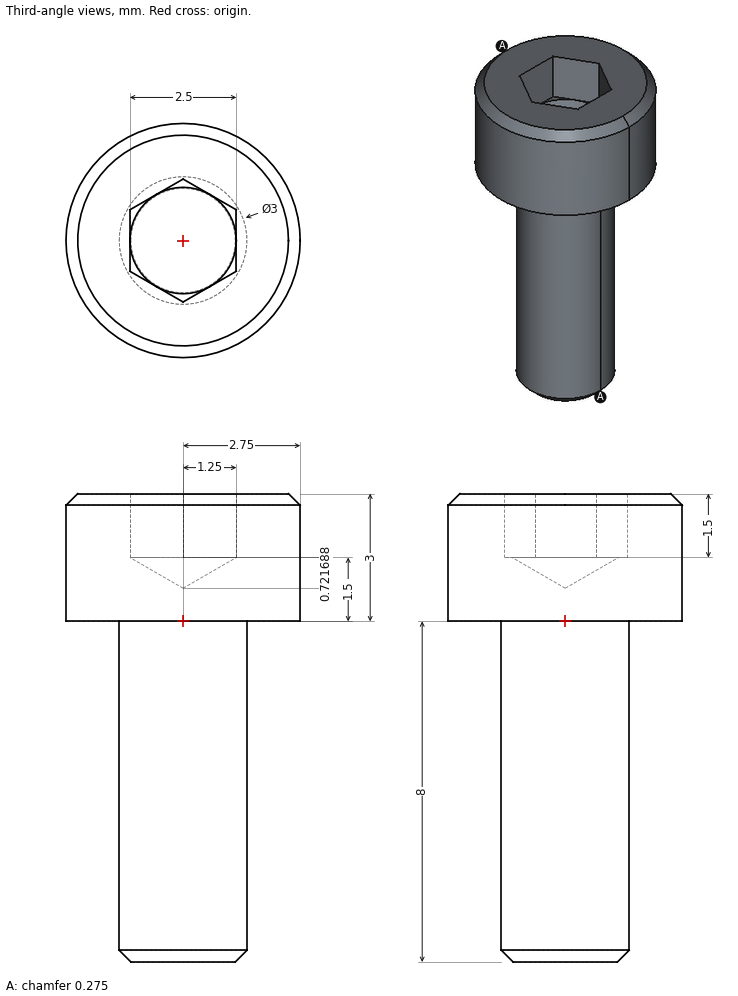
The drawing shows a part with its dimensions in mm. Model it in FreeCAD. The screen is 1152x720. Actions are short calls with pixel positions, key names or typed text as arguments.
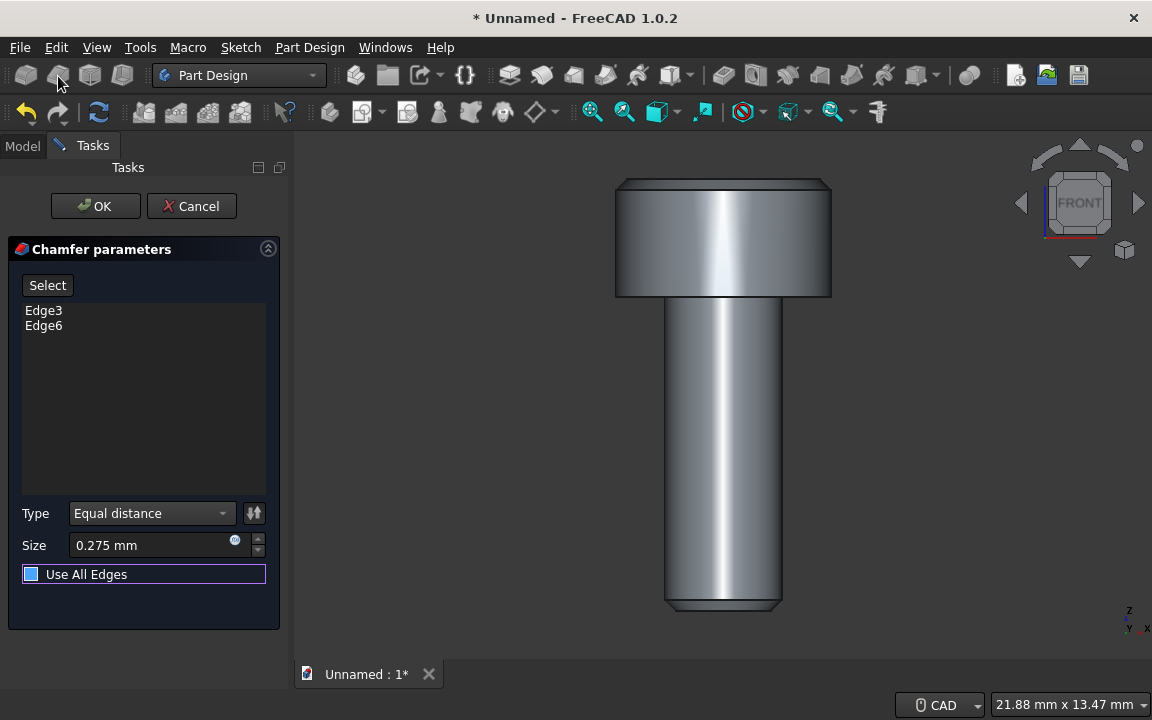
click(96, 206)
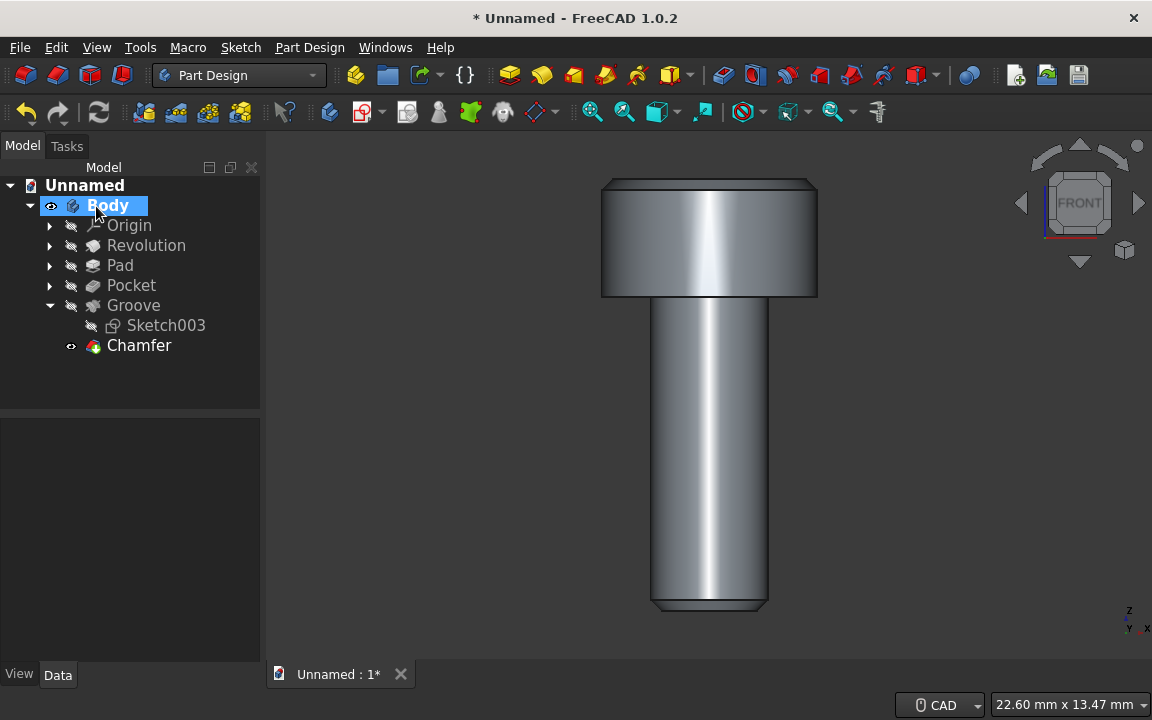
key(0)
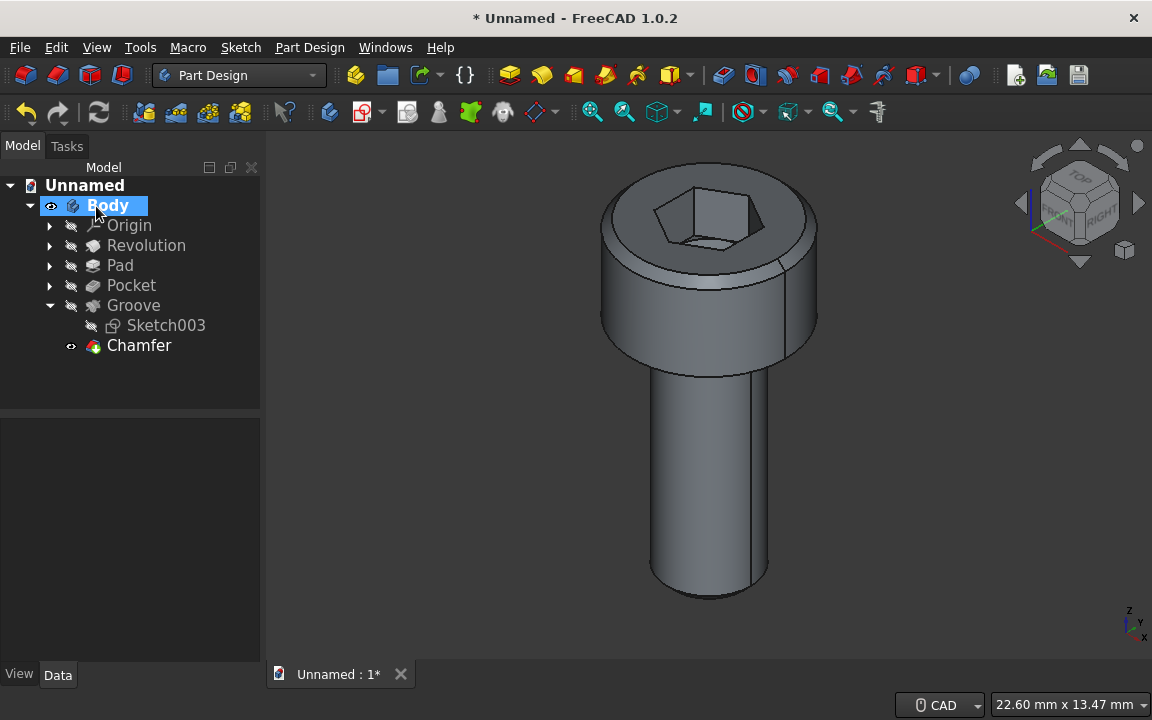
key(v)
key(f)